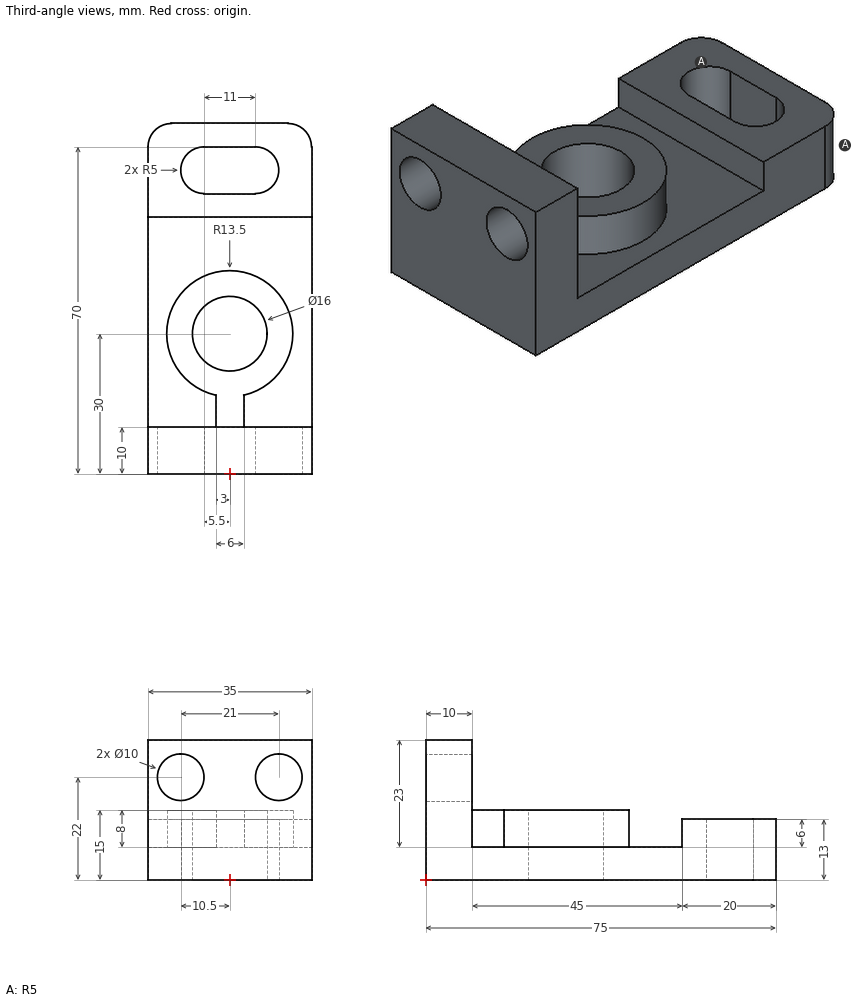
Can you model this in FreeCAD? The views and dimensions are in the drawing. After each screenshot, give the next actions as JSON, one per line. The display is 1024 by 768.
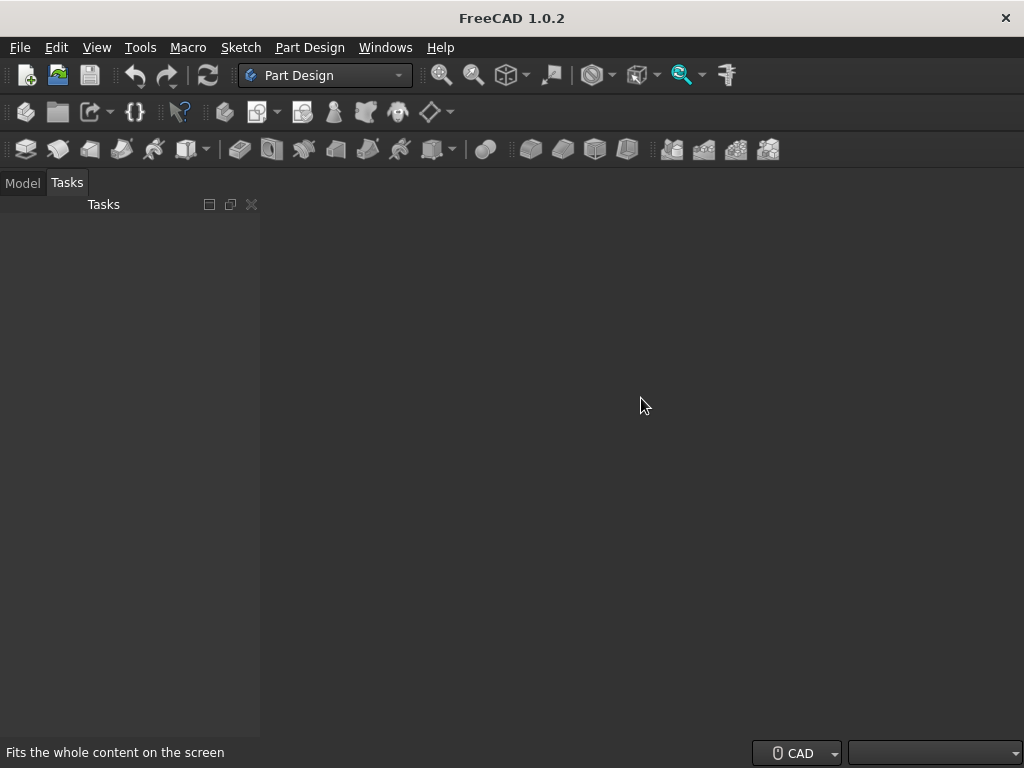
{"action": "key", "text": "ctrl+n"}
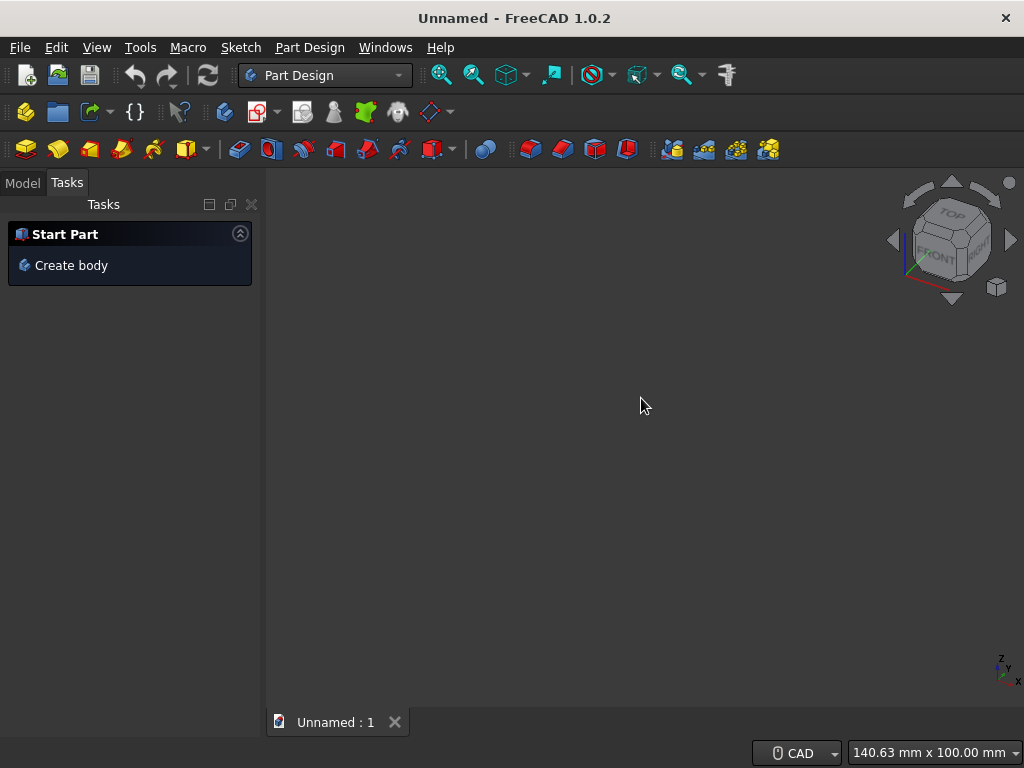
{"action": "left_click", "coordinate": [258, 112]}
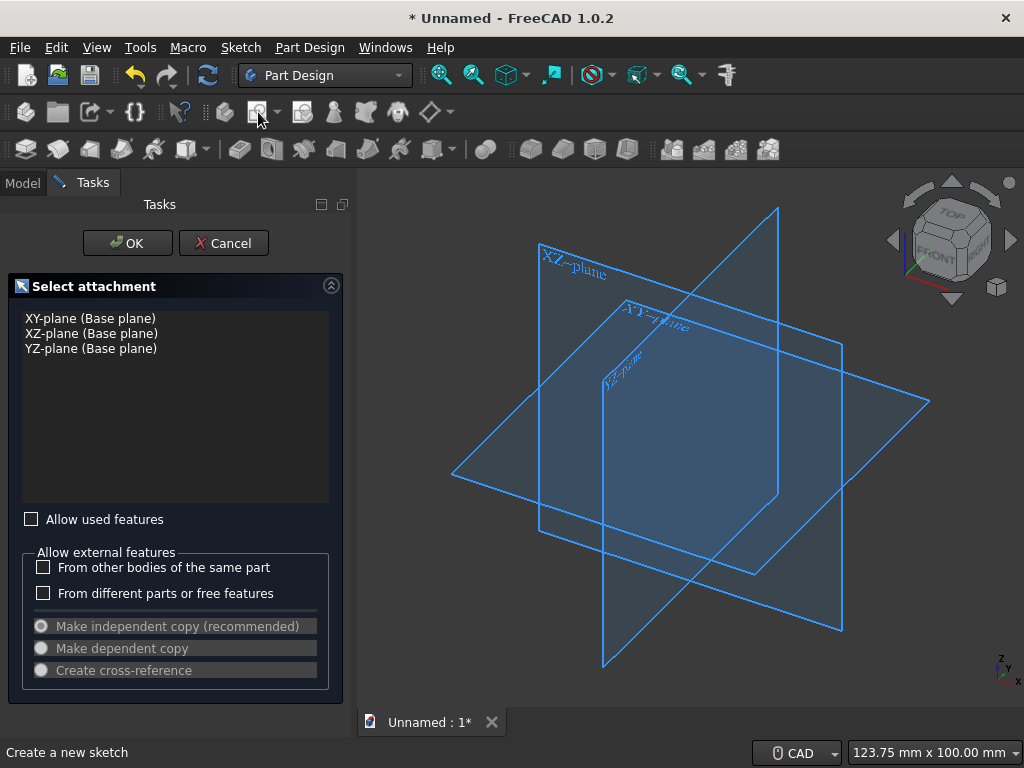
{"action": "left_click", "coordinate": [82, 348]}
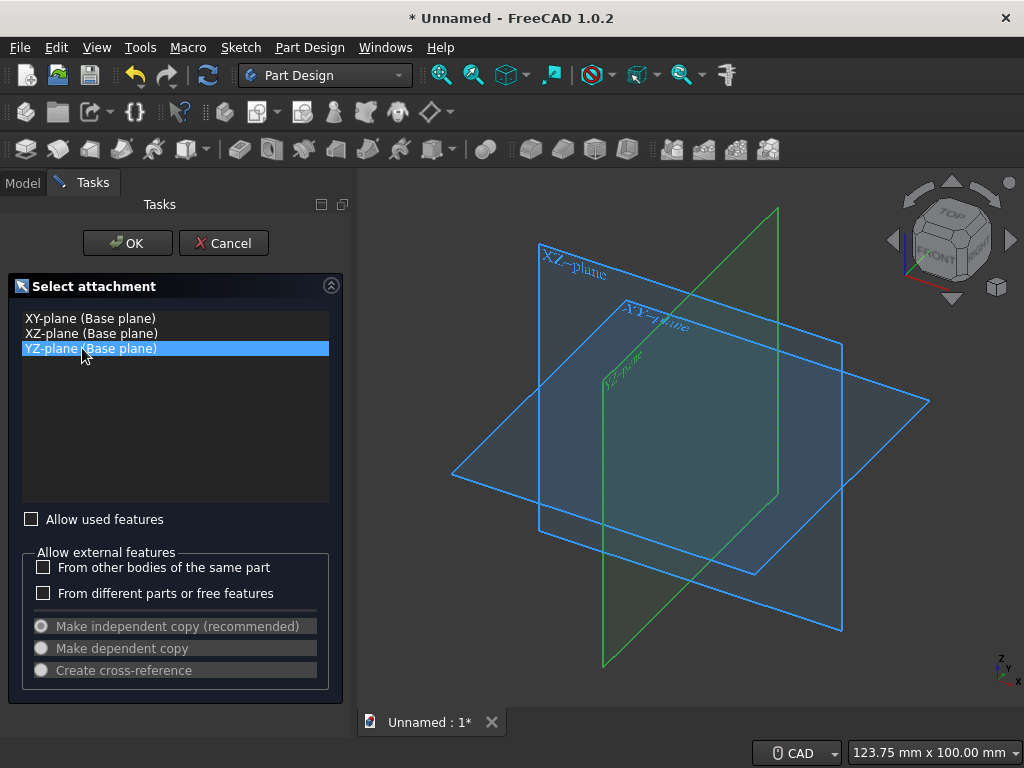
{"action": "left_click", "coordinate": [128, 243]}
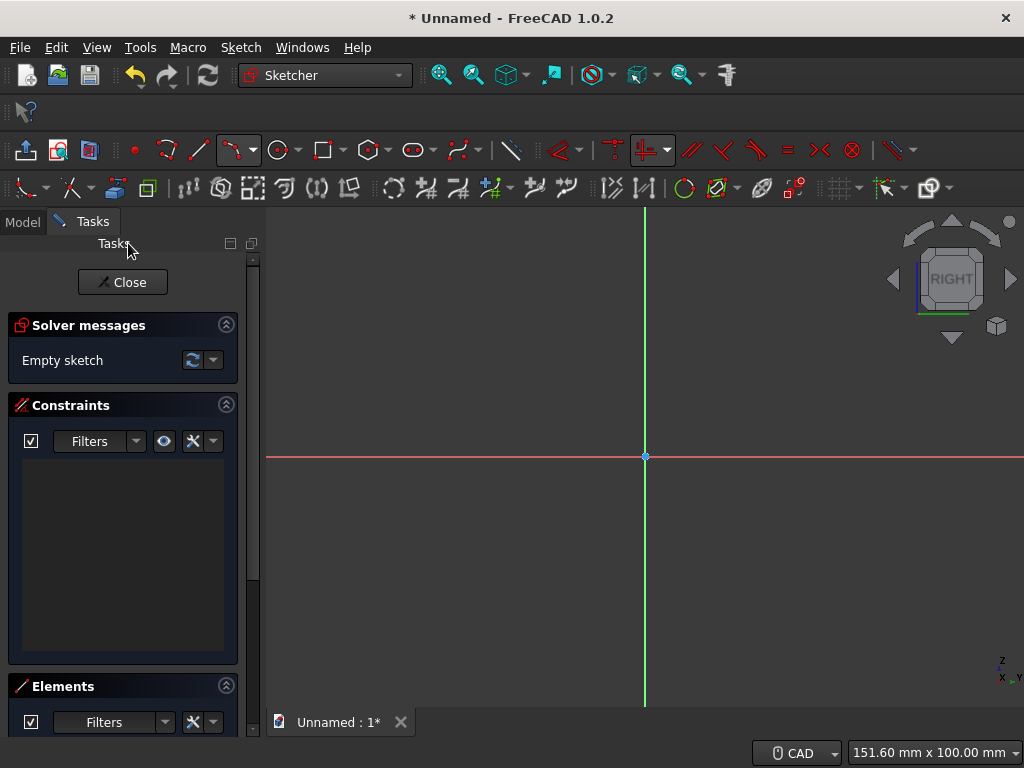
{"action": "scroll", "coordinate": [294, 609], "scroll_direction": "down", "scroll_amount": 2}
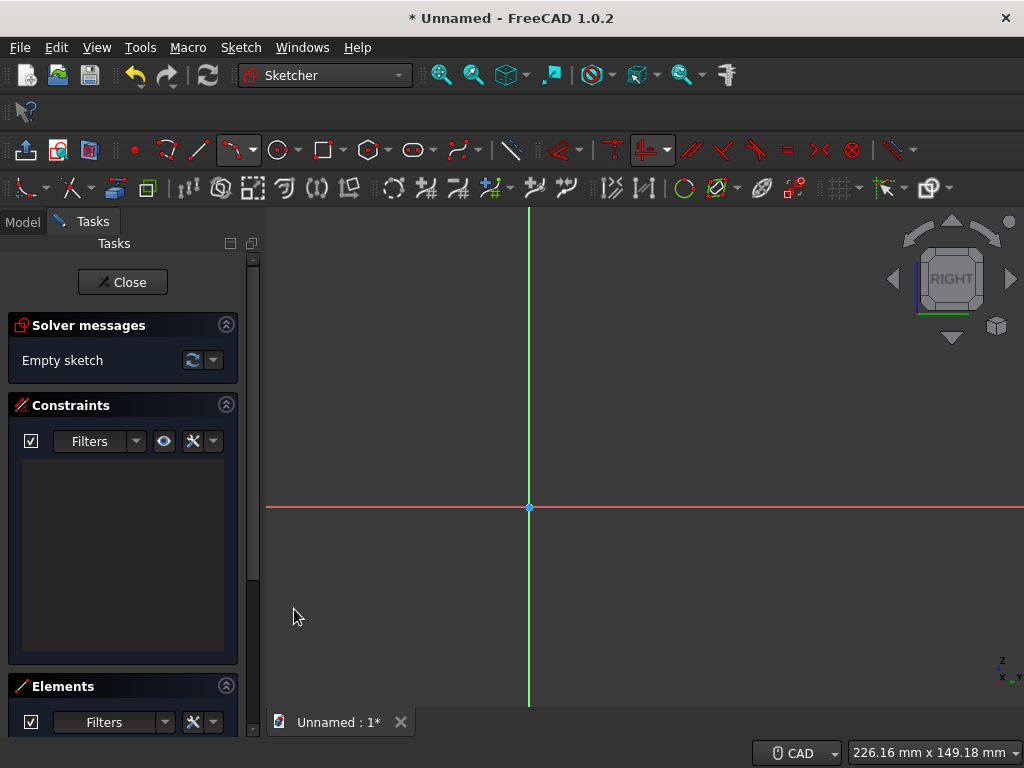
{"action": "scroll", "coordinate": [815, 457], "scroll_direction": "up", "scroll_amount": 2}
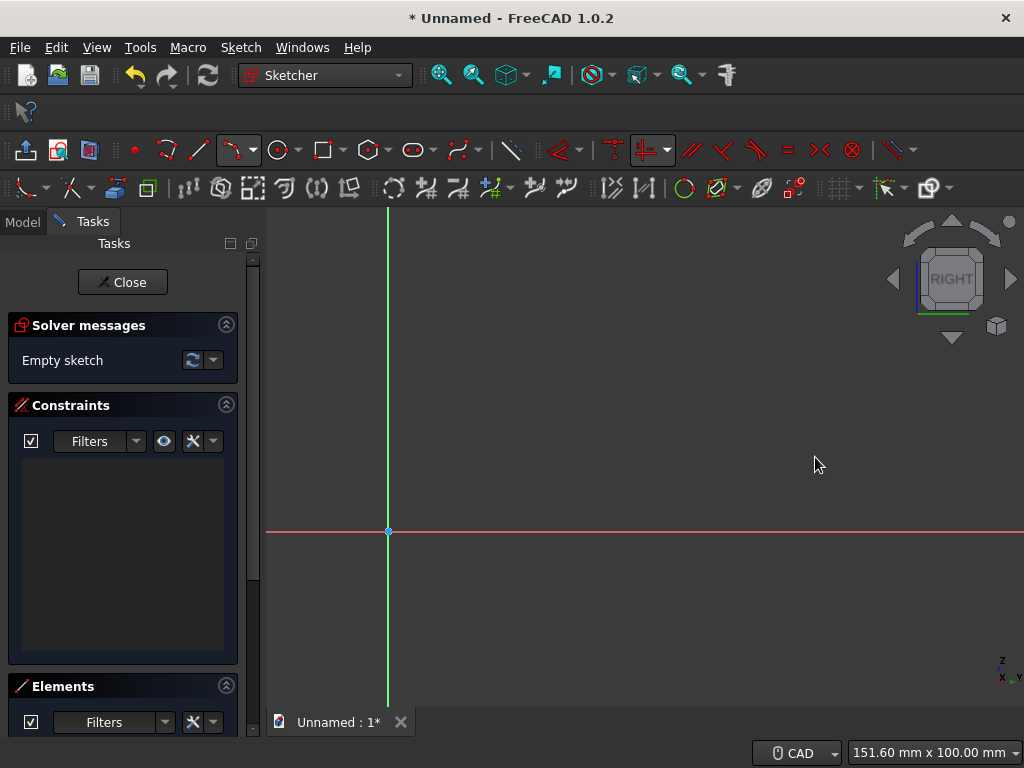
{"action": "key", "text": "g m"}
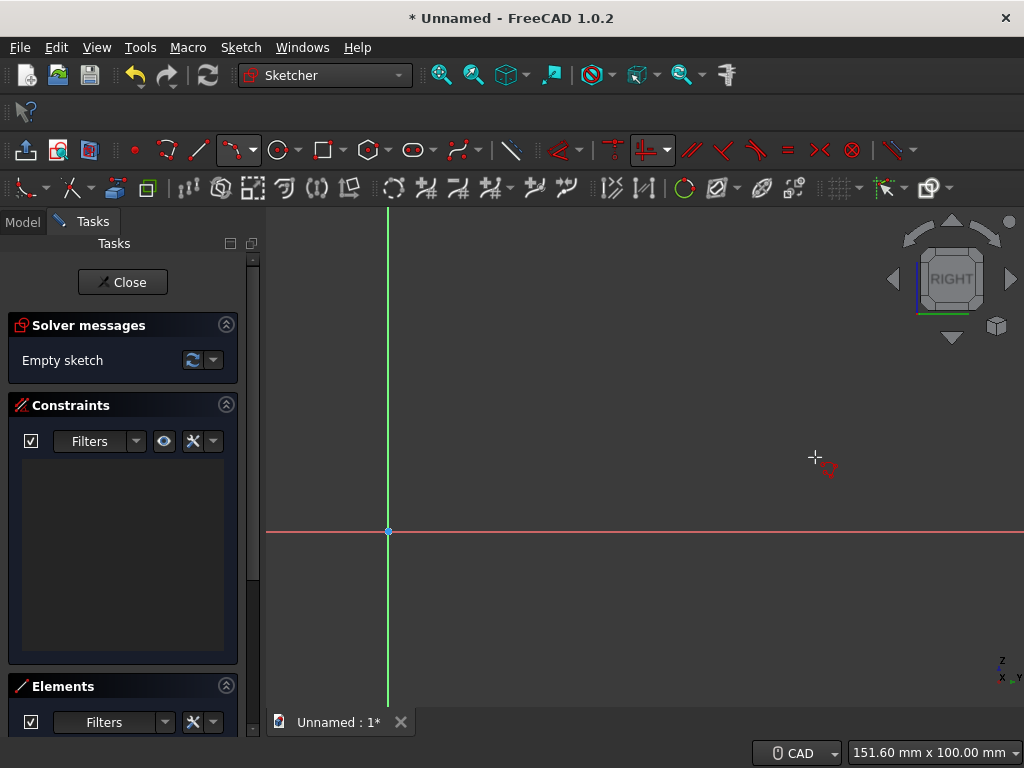
{"action": "left_click", "coordinate": [388, 532]}
{"action": "left_click", "coordinate": [763, 523]}
{"action": "left_click", "coordinate": [763, 467]}
{"action": "left_click", "coordinate": [663, 467]}
{"action": "left_click", "coordinate": [663, 497]}
{"action": "left_click", "coordinate": [438, 497]}
{"action": "left_click", "coordinate": [438, 382]}
{"action": "left_click", "coordinate": [397, 382]}
{"action": "left_click", "coordinate": [388, 532]}
{"action": "key", "text": "Escape"}
{"action": "key", "text": "Escape"}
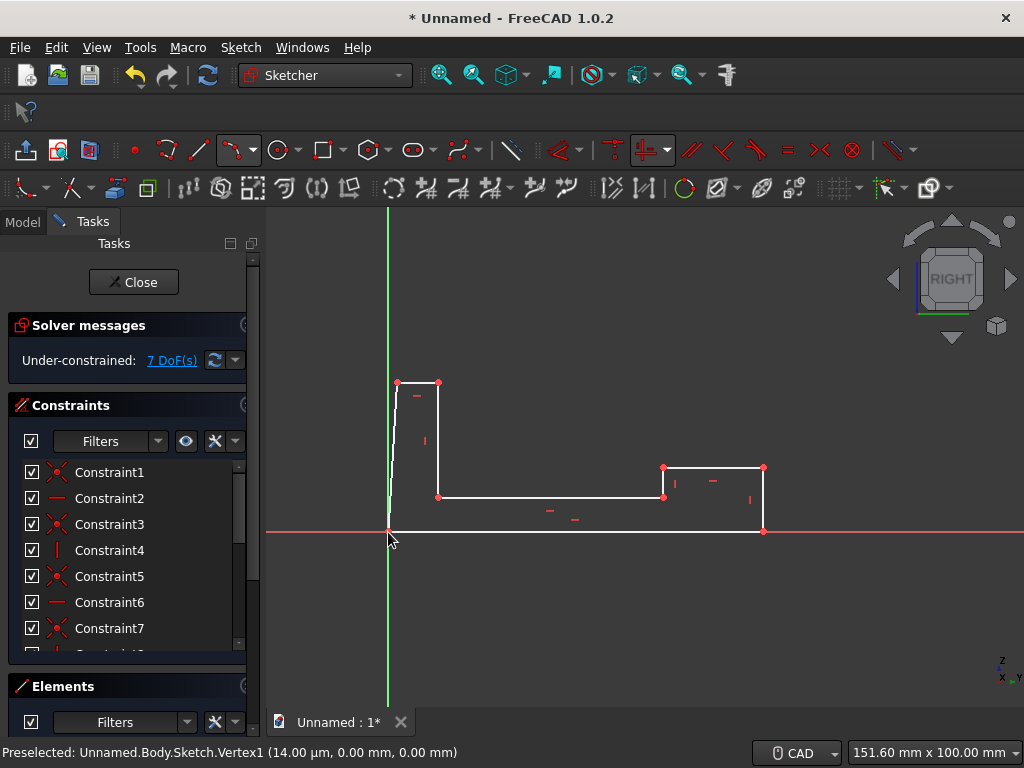
{"action": "left_click", "coordinate": [391, 487]}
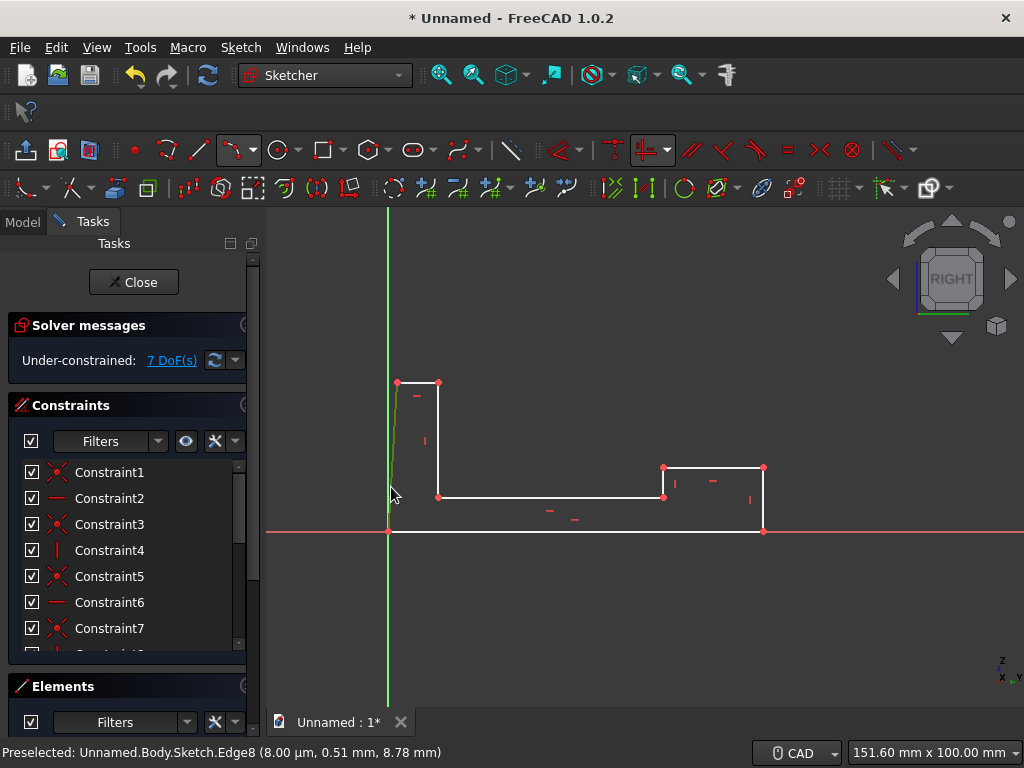
{"action": "key", "text": "v"}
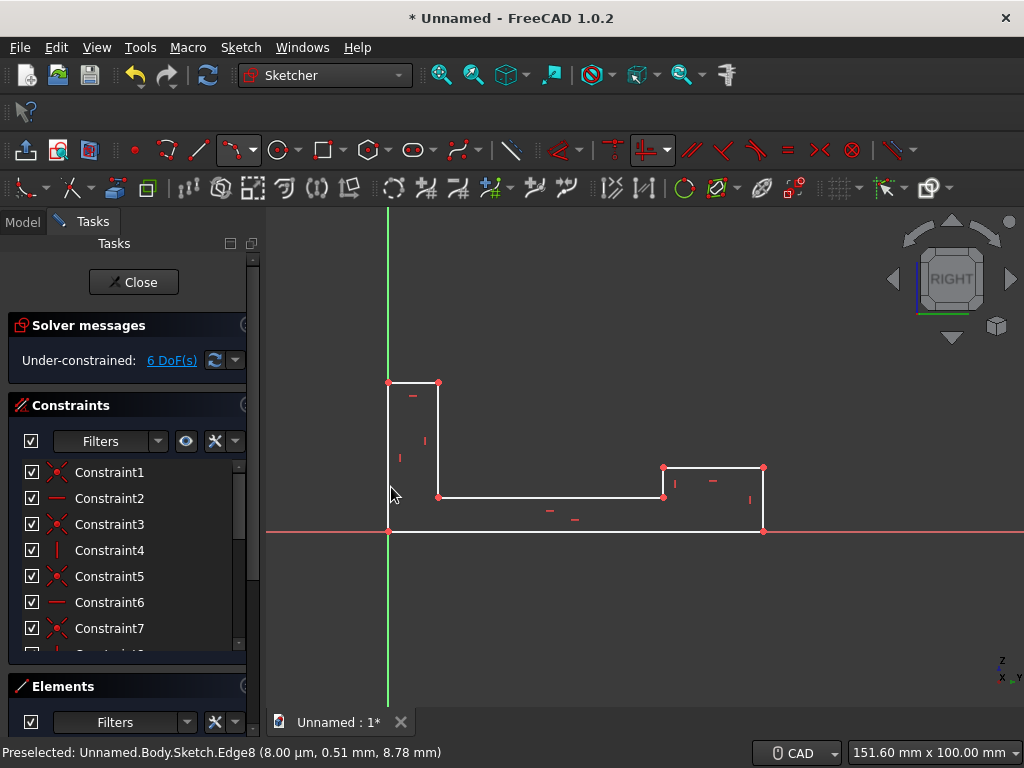
{"action": "key", "text": "d"}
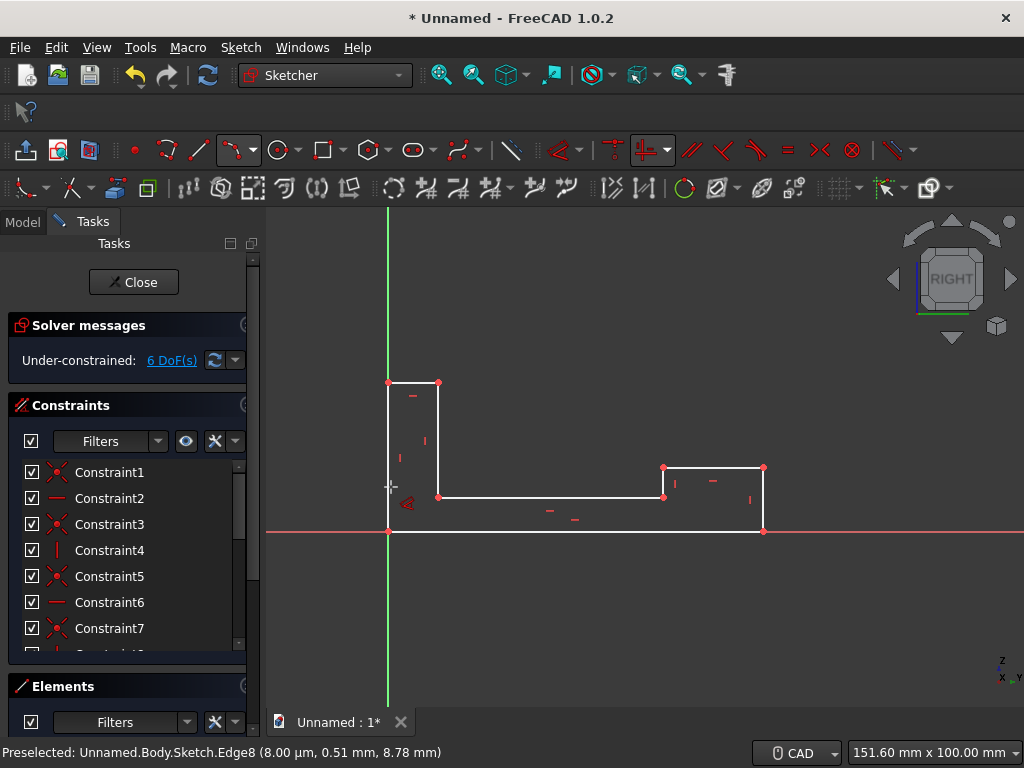
{"action": "scroll", "coordinate": [663, 480], "scroll_direction": "up", "scroll_amount": 2}